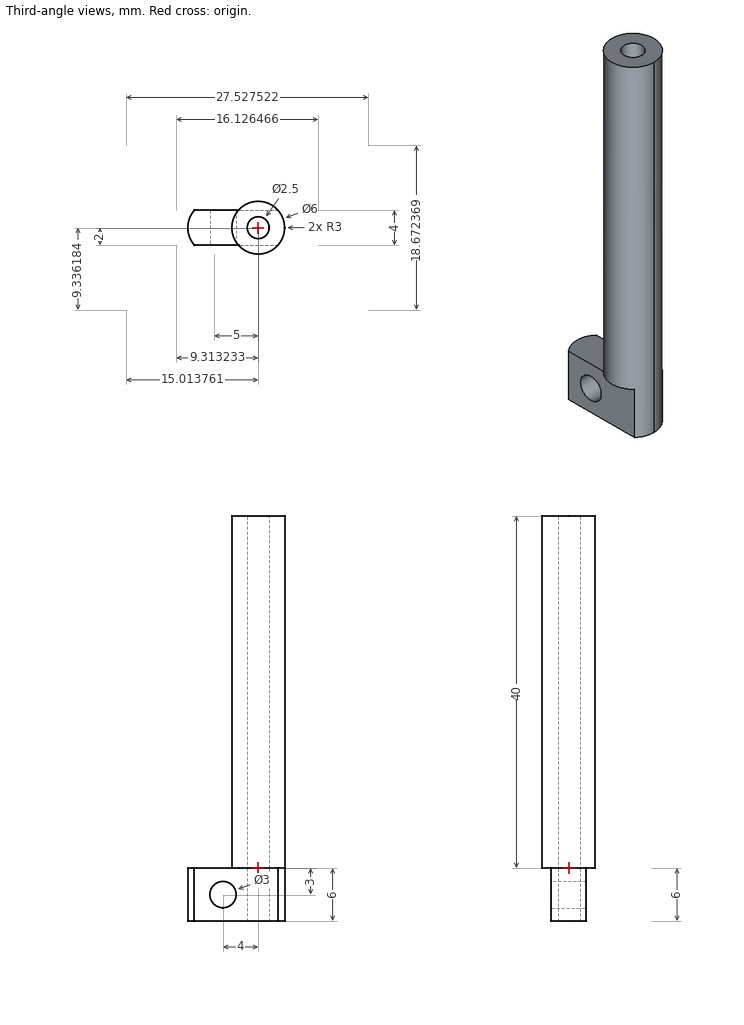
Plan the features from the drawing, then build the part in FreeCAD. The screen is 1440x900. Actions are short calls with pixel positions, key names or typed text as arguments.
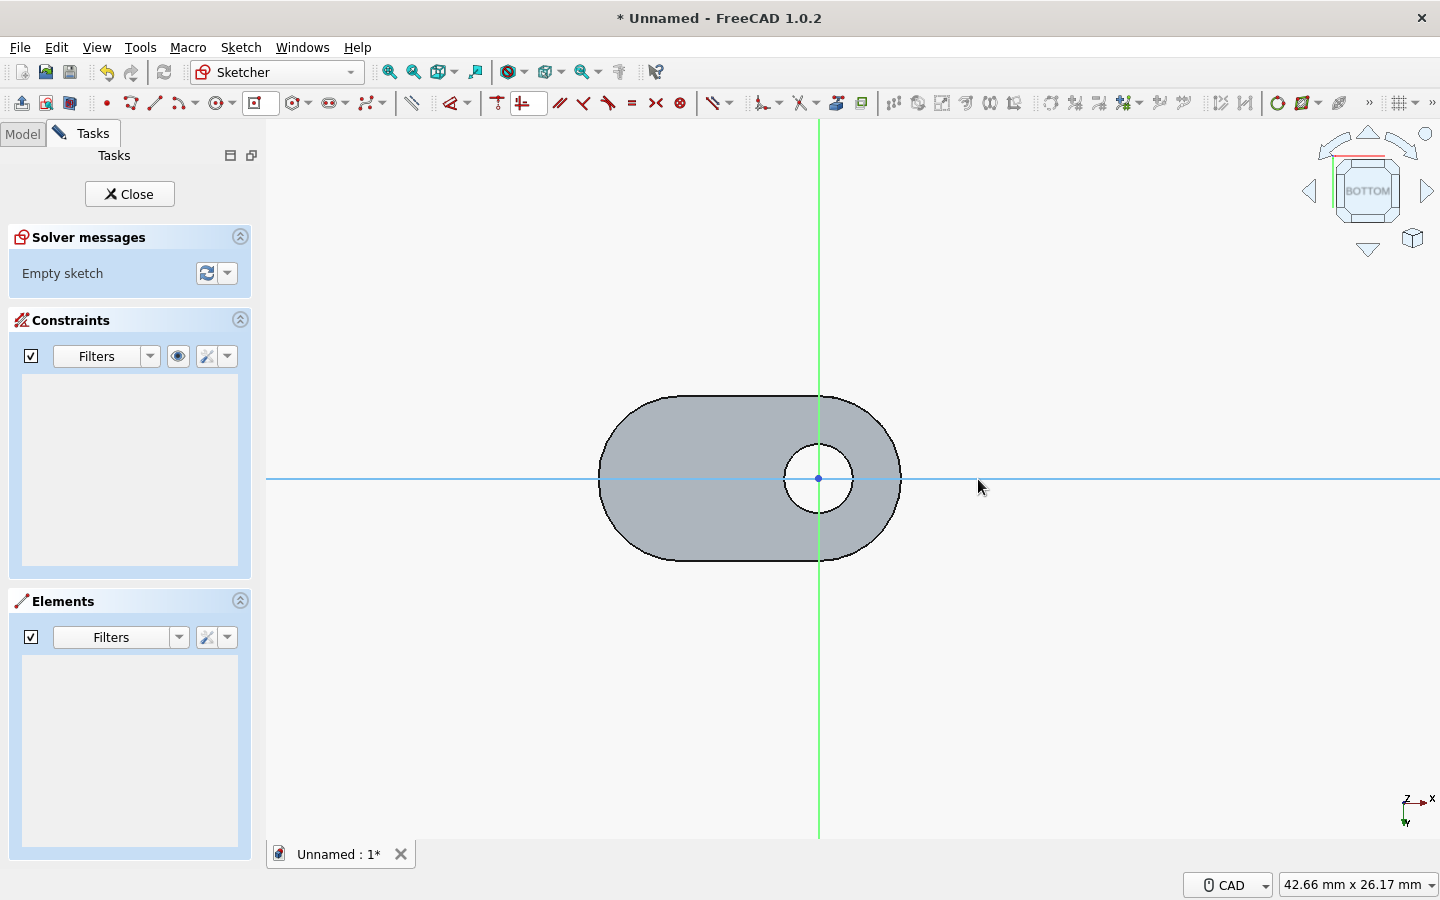
key(g)
key(r)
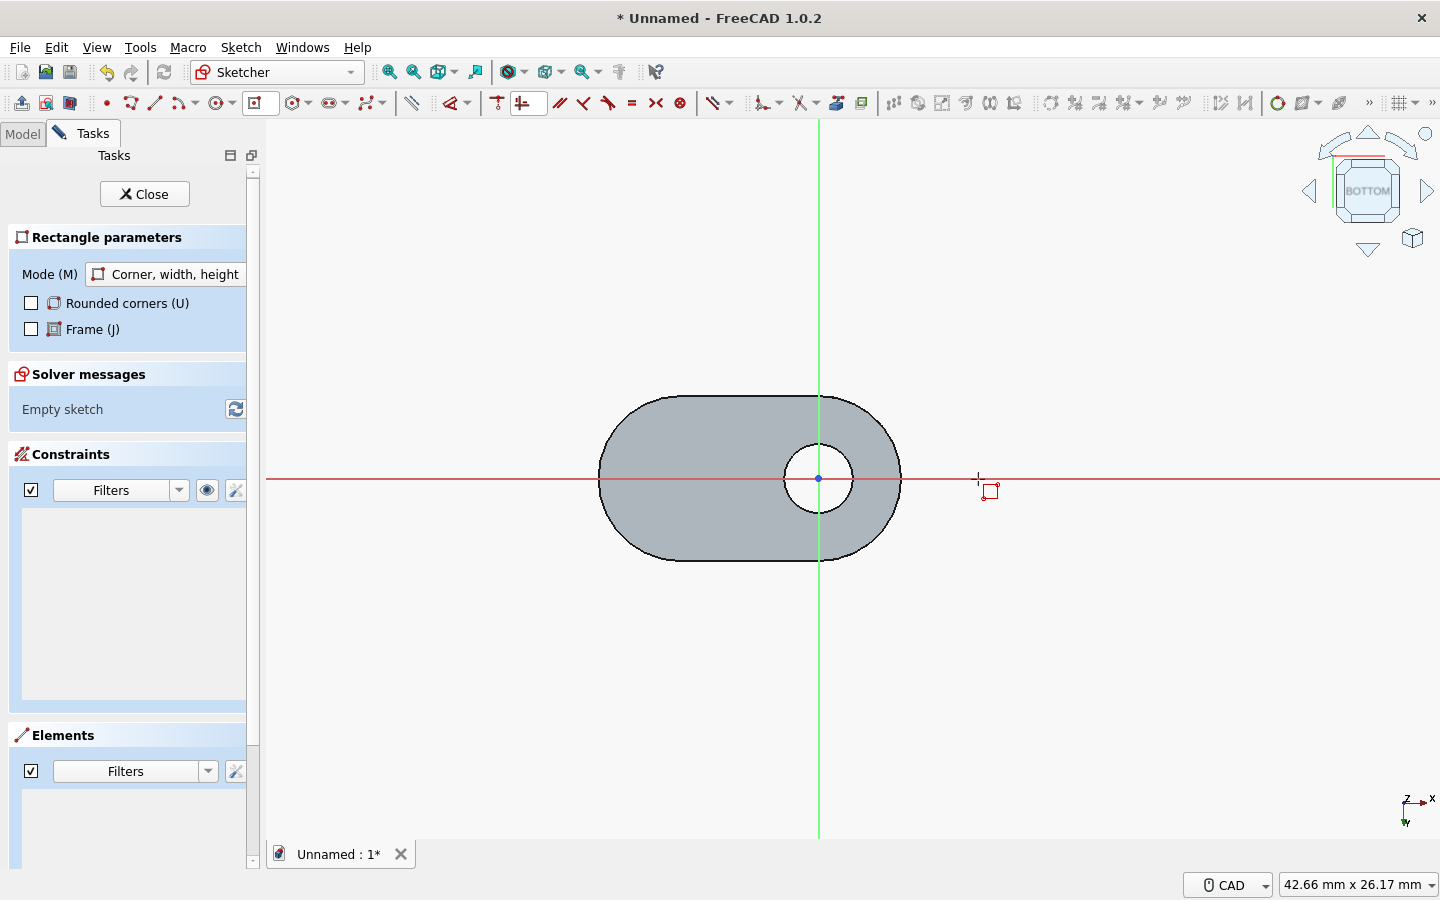
click(405, 222)
move(1163, 735)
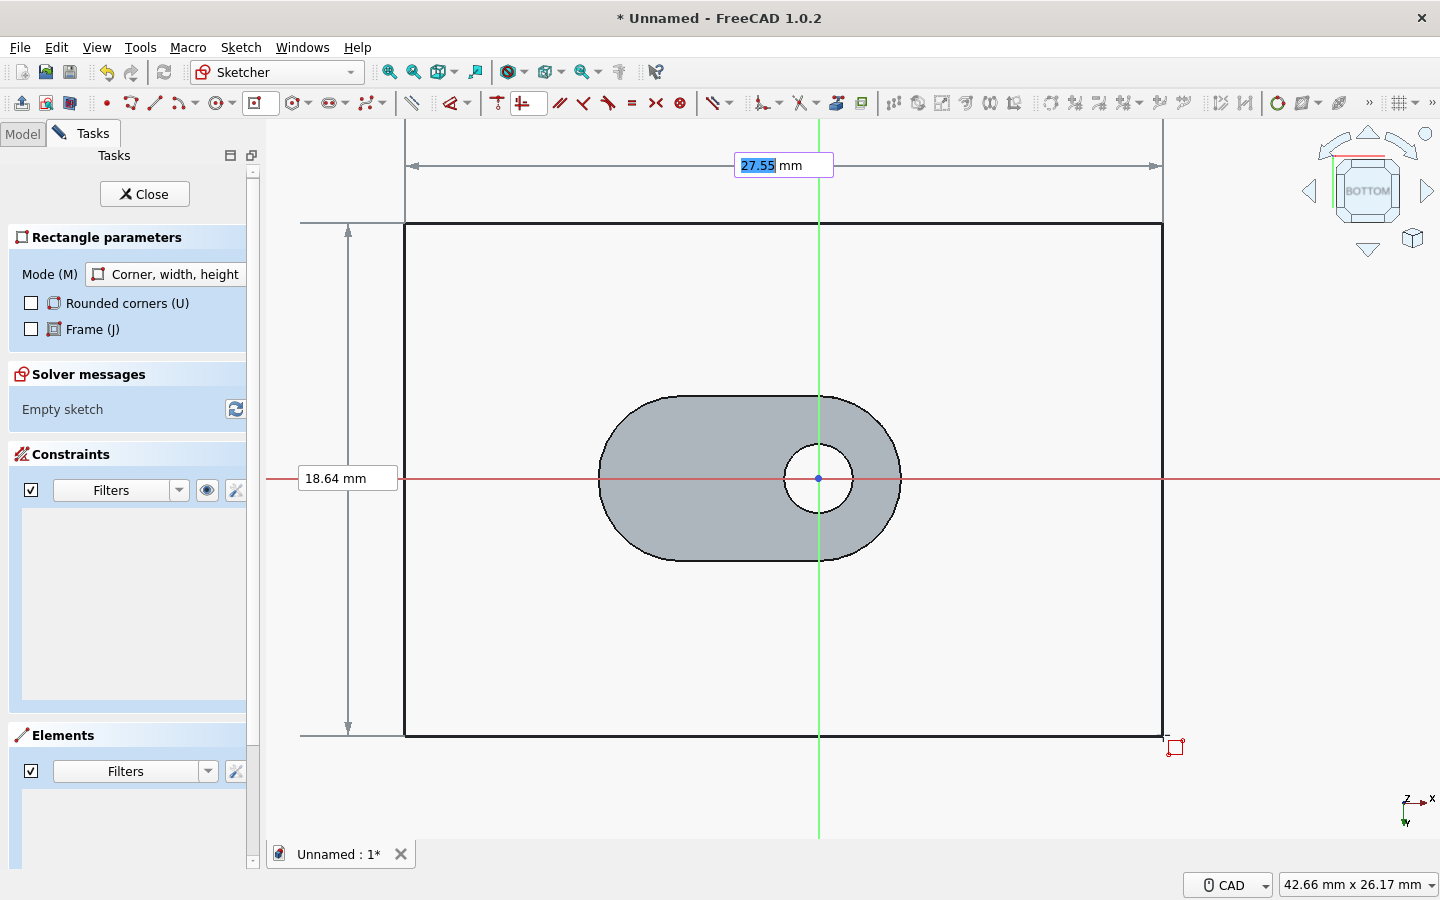
text(27.527522)
key(Tab)
text(18.672369)
key(Return)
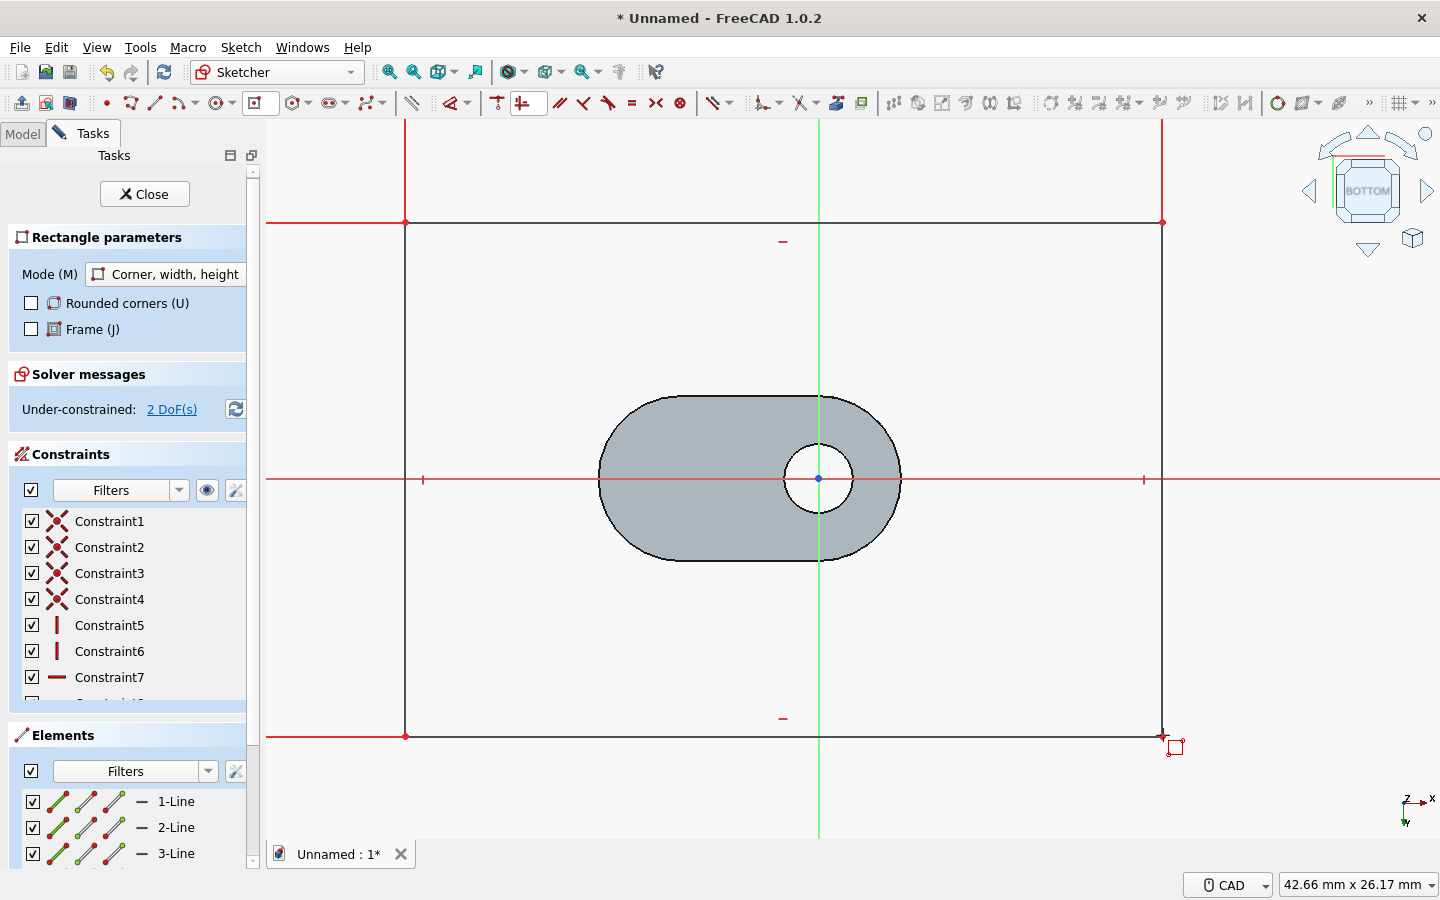
click(562, 424)
move(1006, 534)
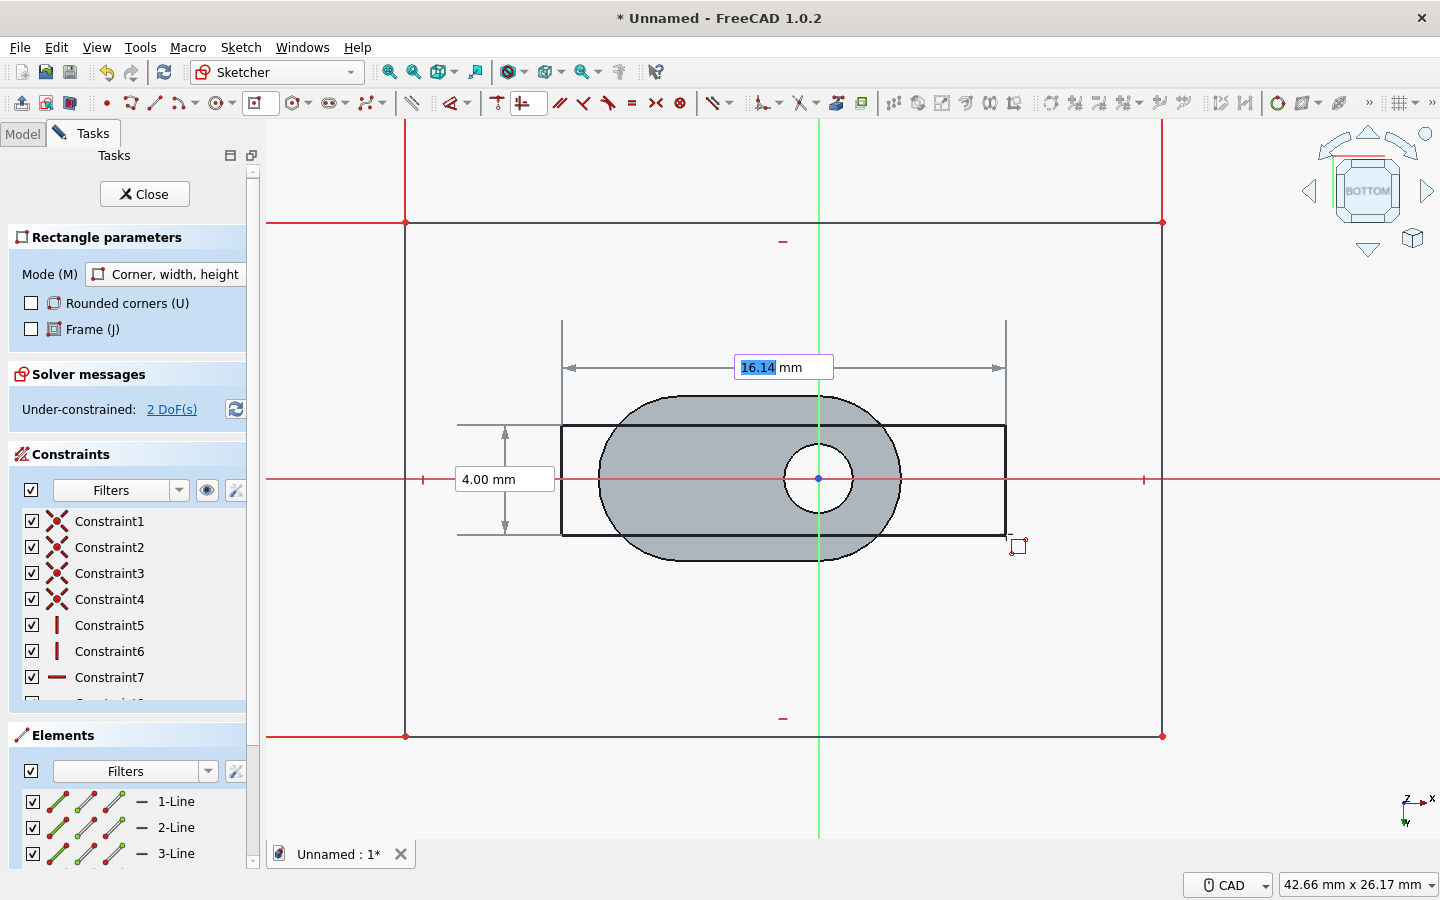
text(16.126466)
key(Tab)
text(4)
key(Return)
key(Escape)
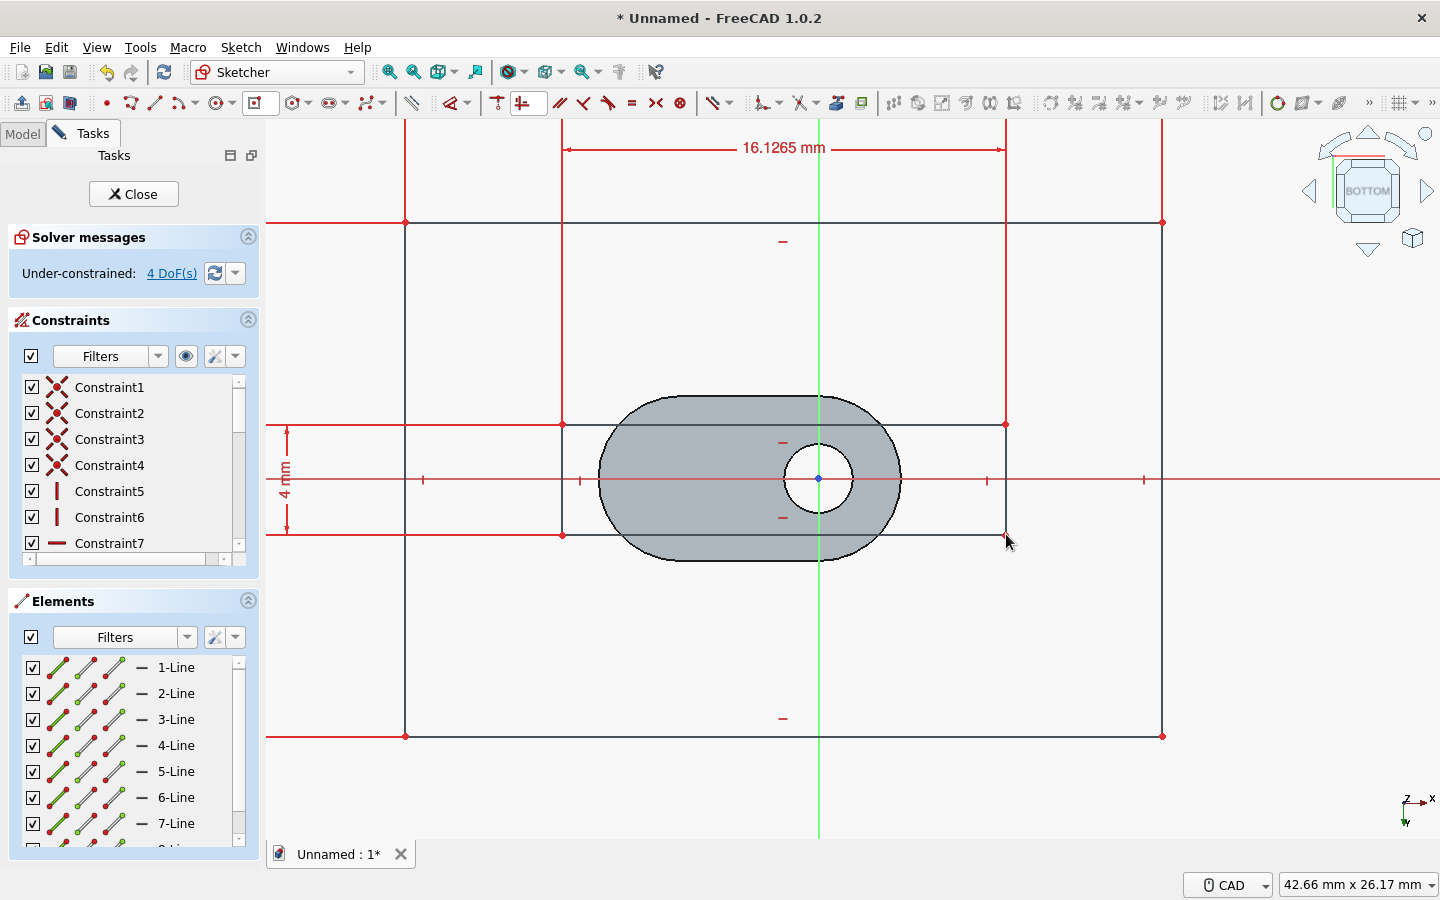
key(d)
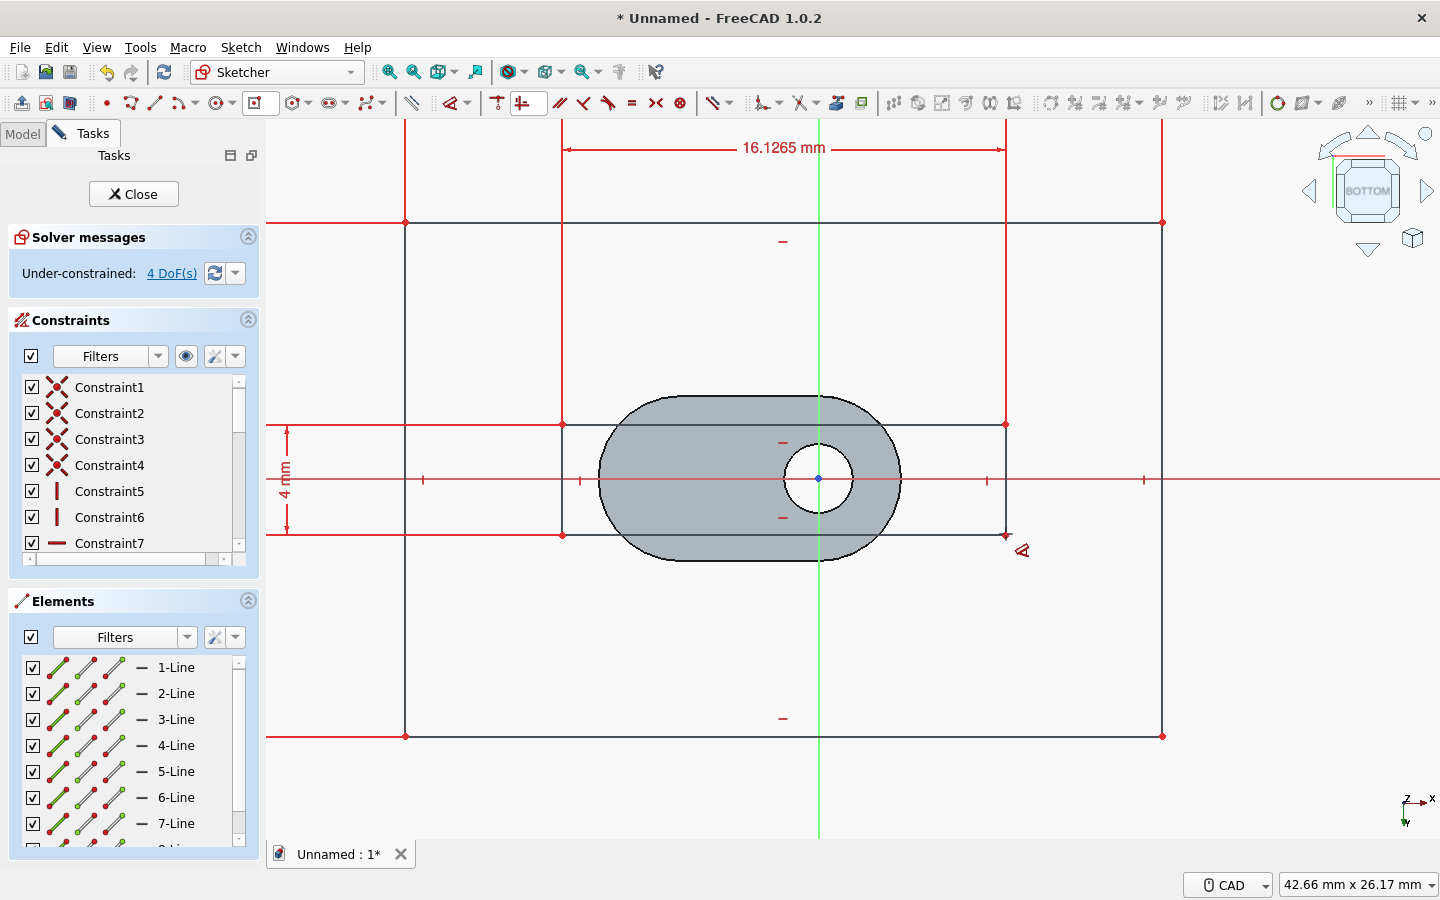
click(562, 425)
click(528, 452)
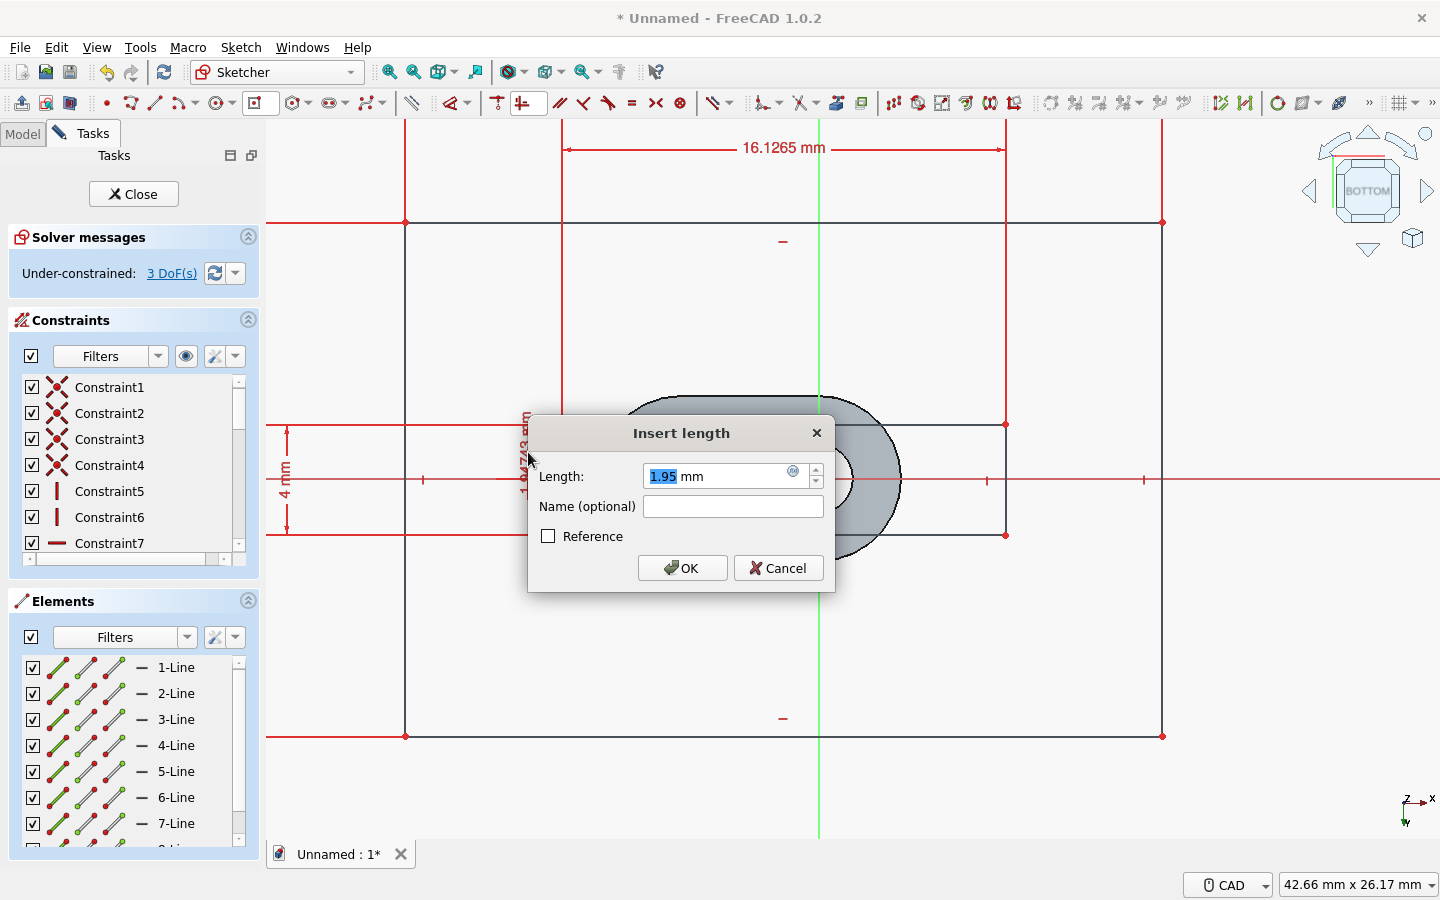
text(2)
key(Return)